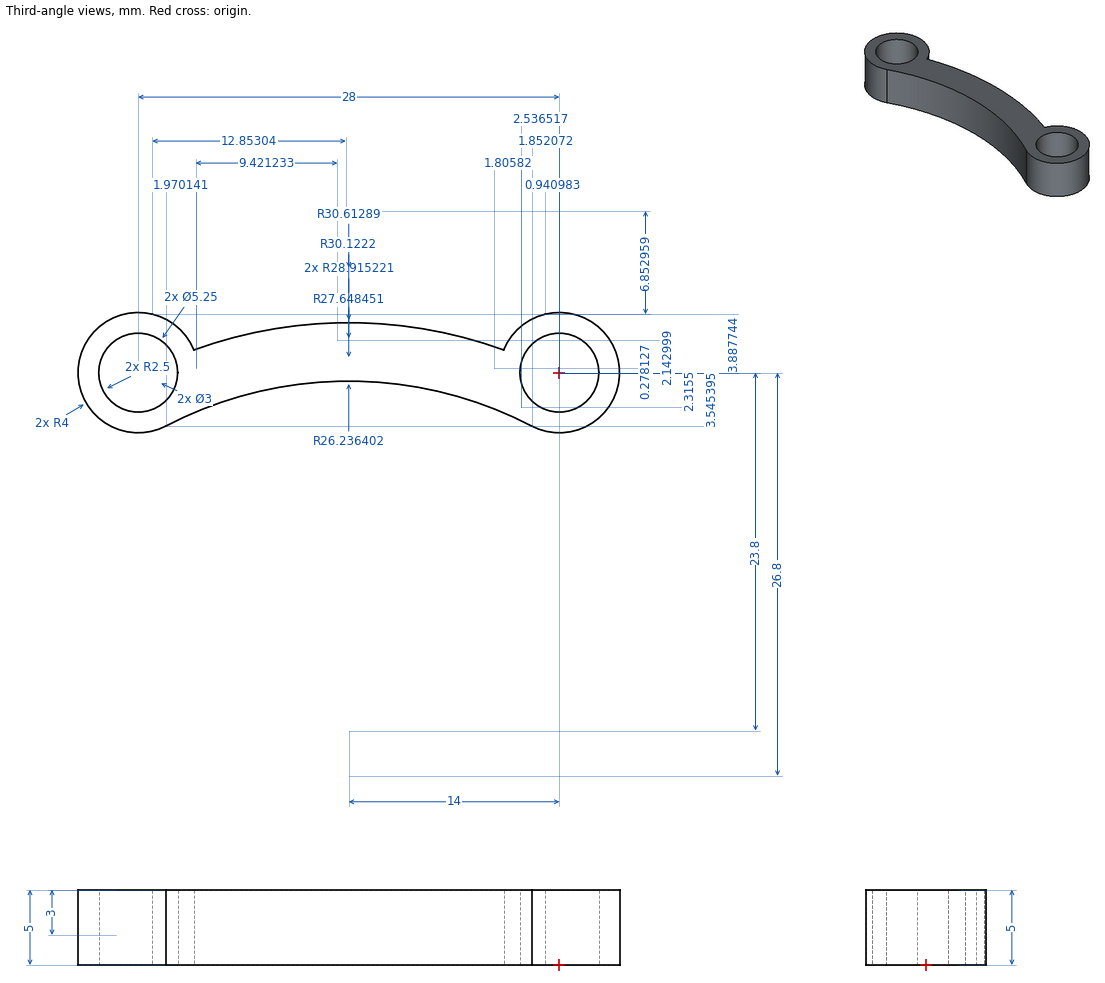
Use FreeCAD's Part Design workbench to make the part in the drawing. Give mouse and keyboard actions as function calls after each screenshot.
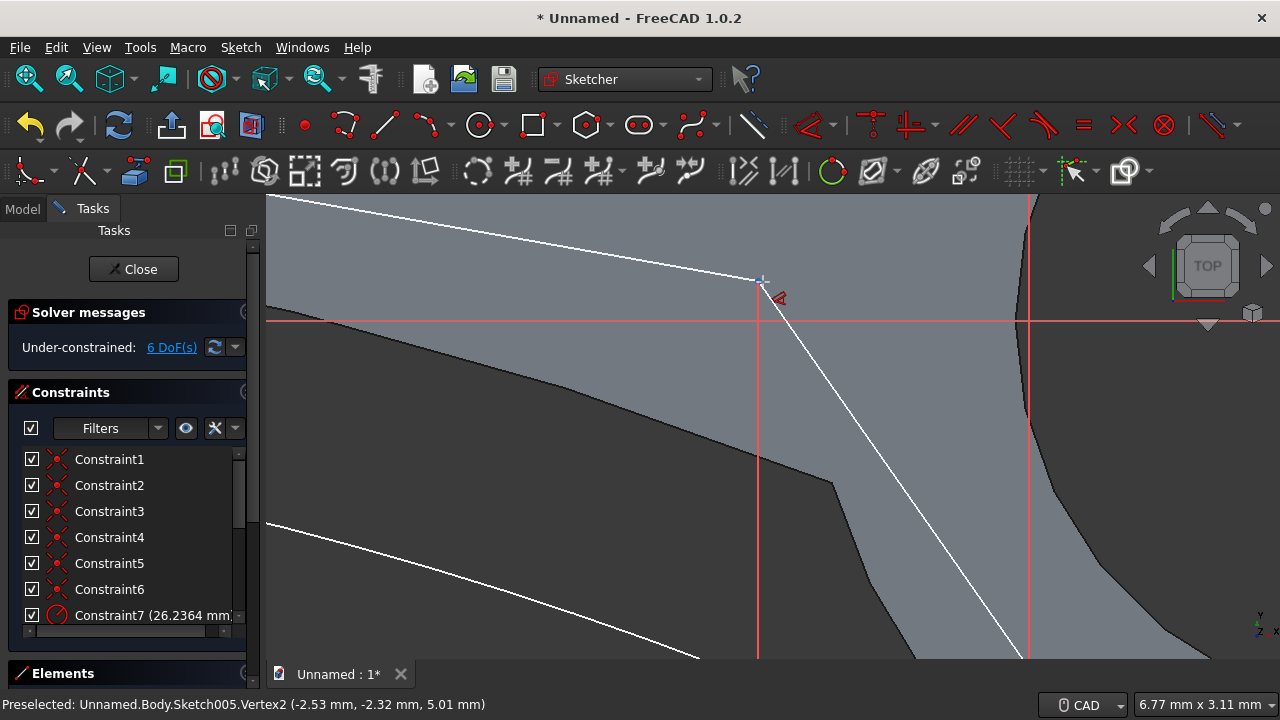
click(758, 281)
click(724, 301)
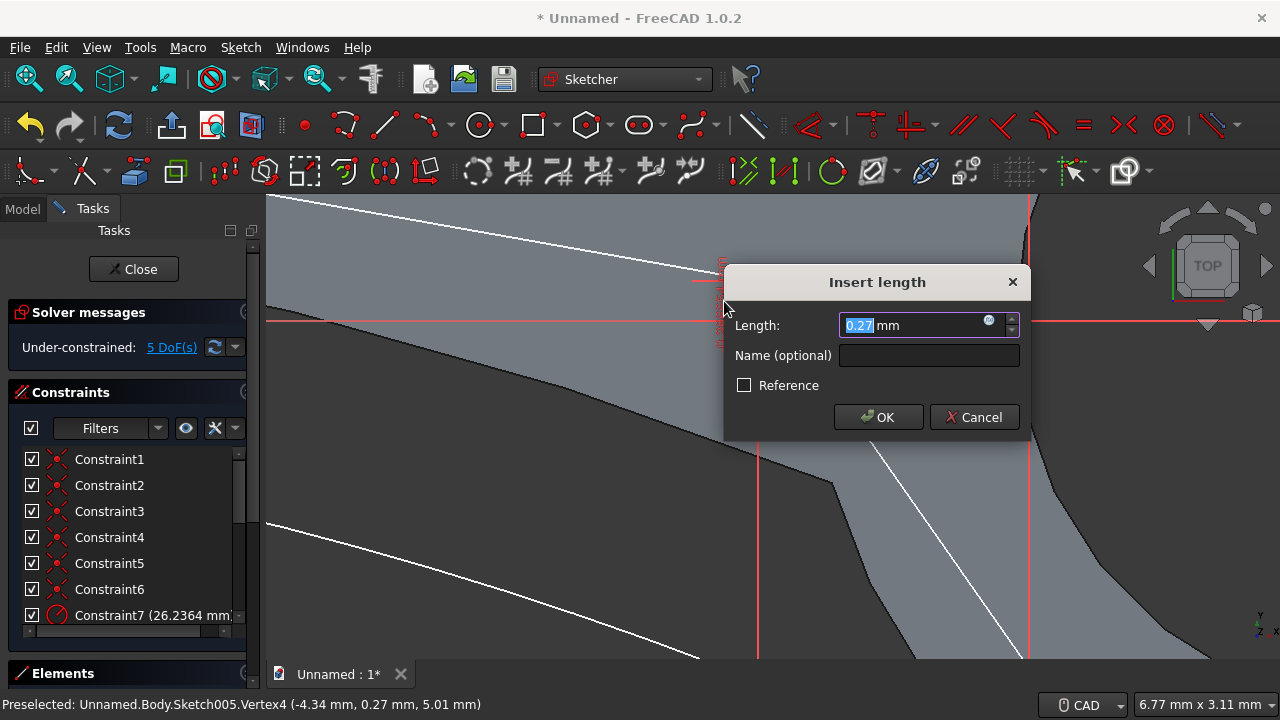
text(0.278127)
key(Return)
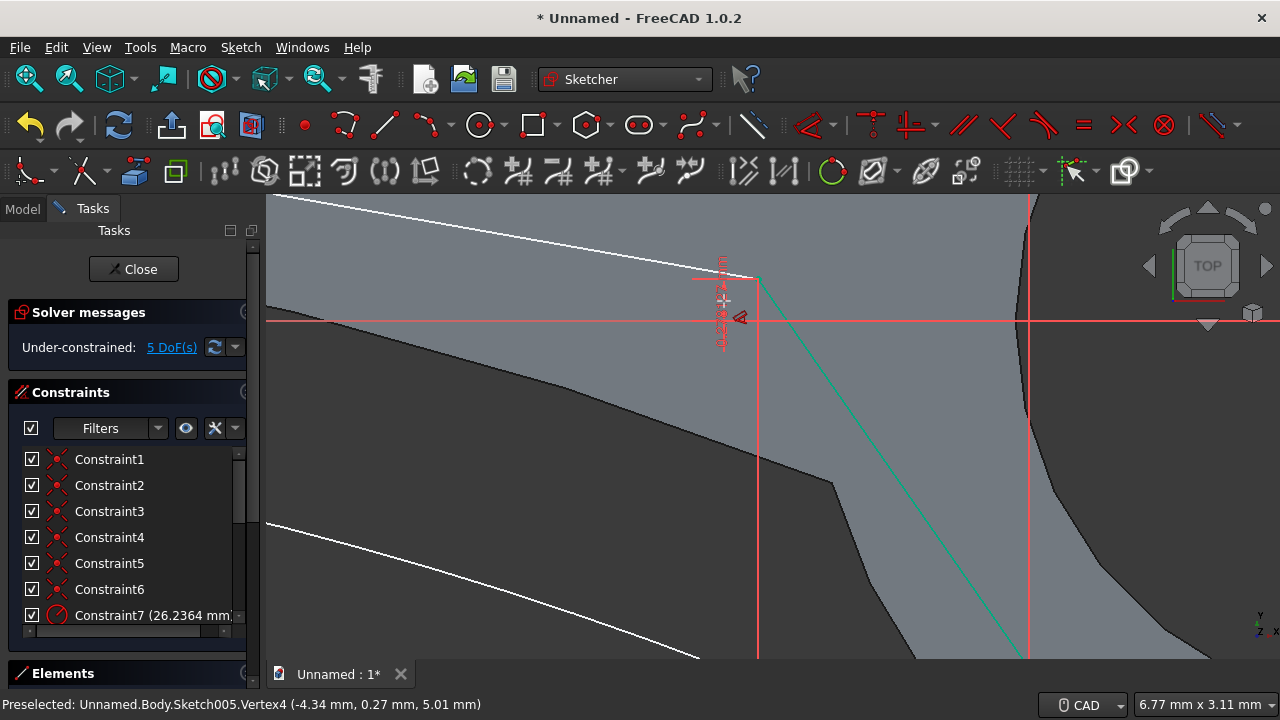
scroll(901, 427, down, 10)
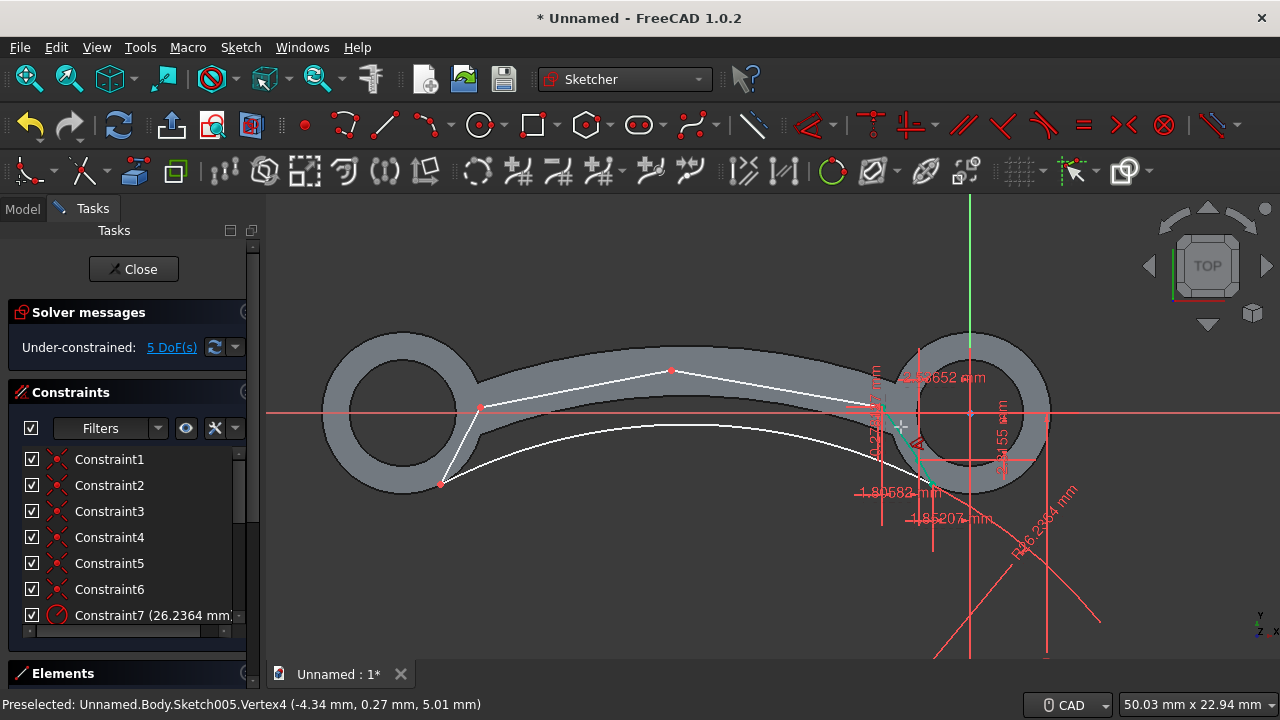
click(671, 370)
click(637, 392)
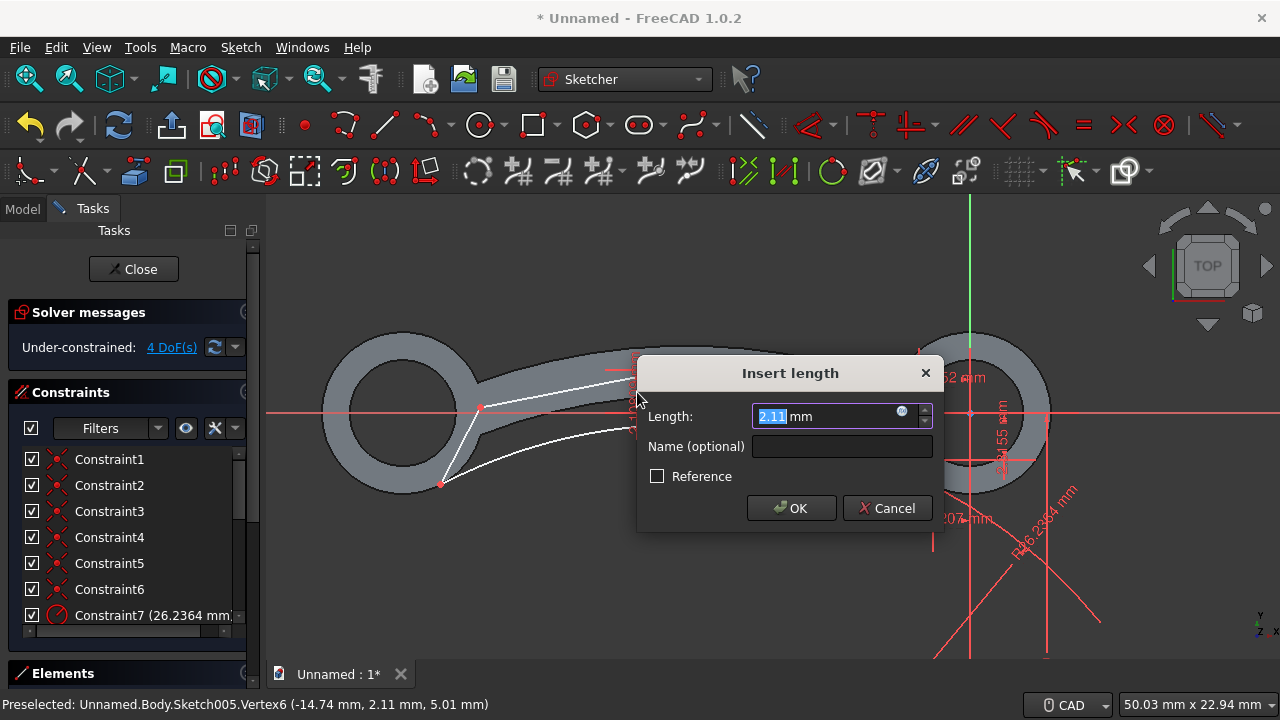
text(2.142999)
key(Return)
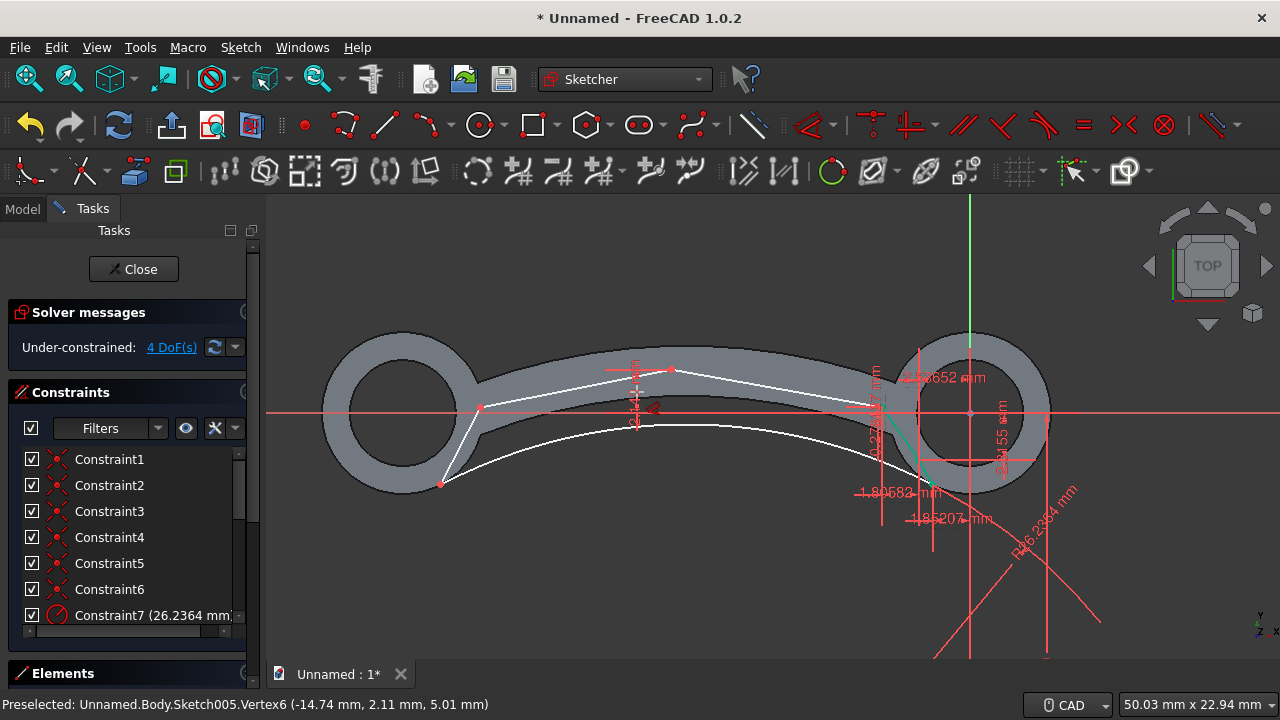
scroll(480, 408, up, 10)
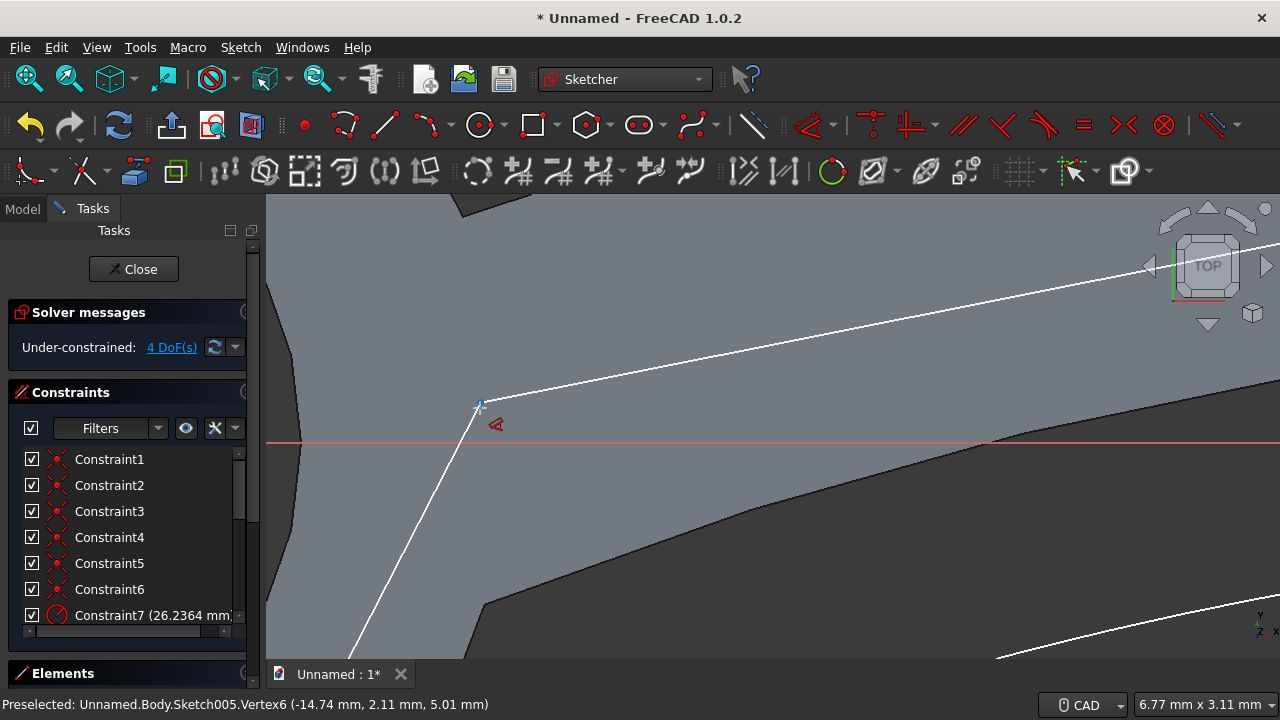
click(481, 403)
click(447, 423)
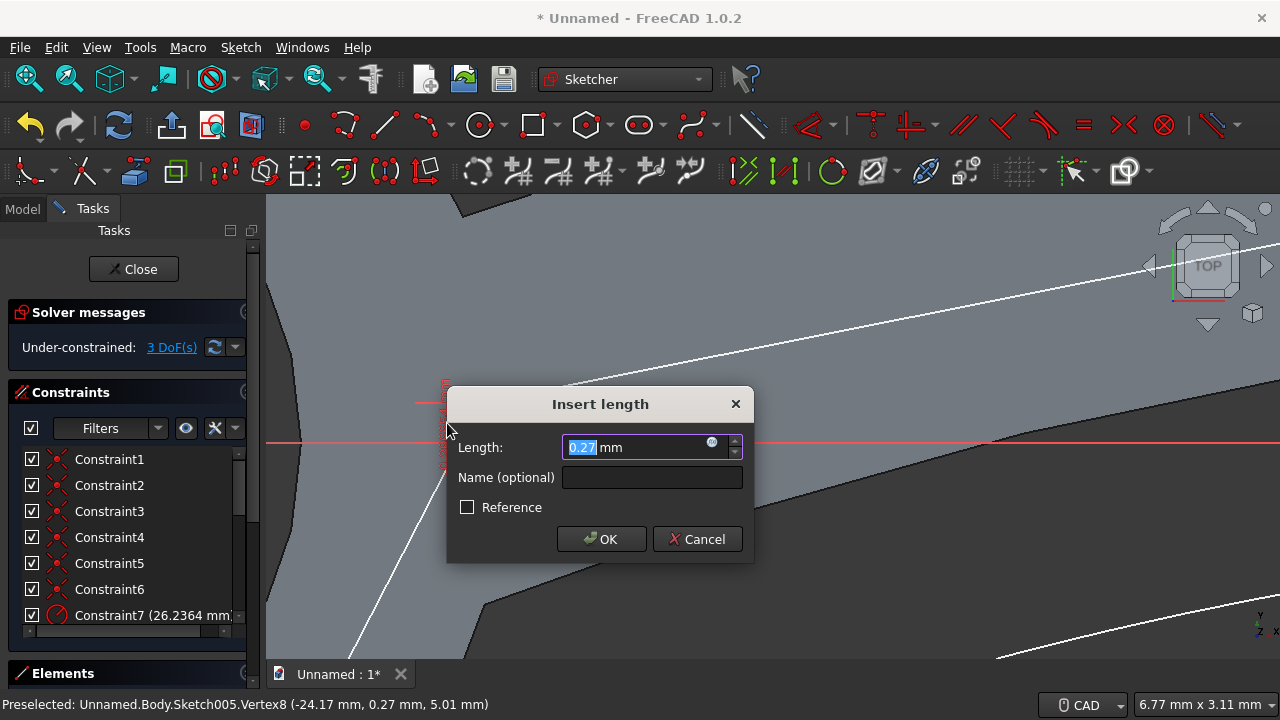
text(0.278127)
key(Return)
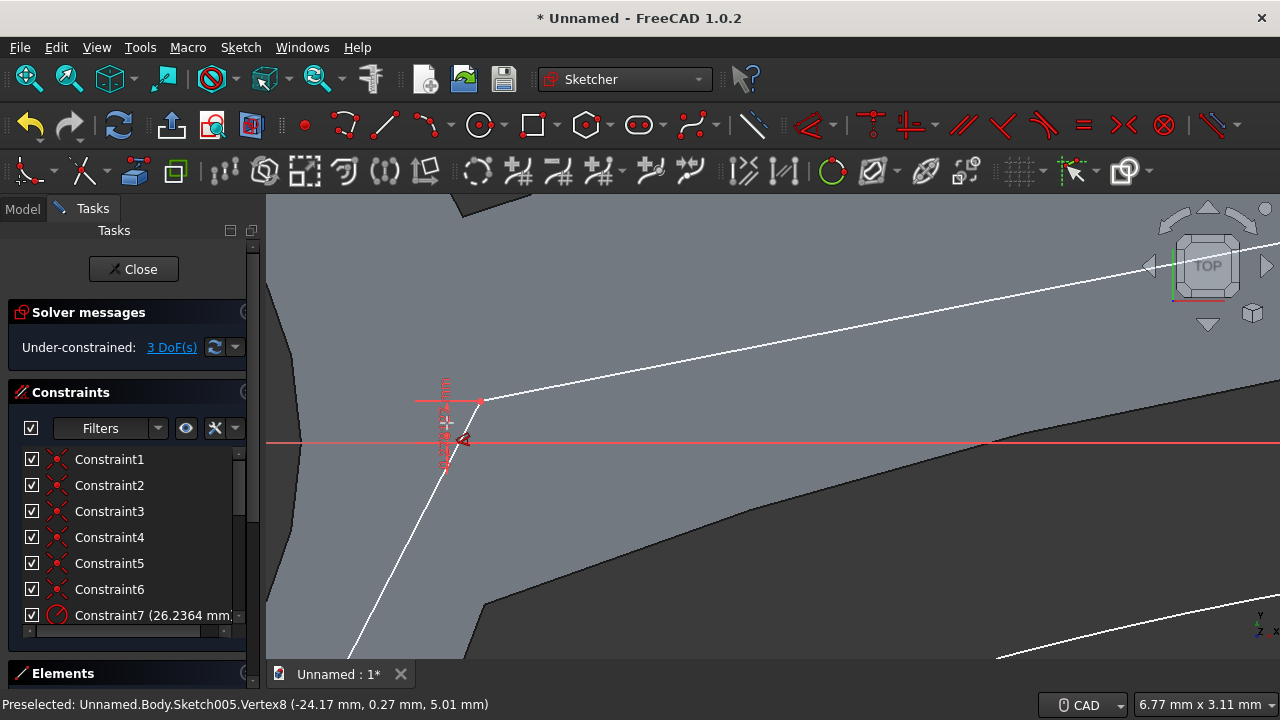
scroll(479, 408, down, 10)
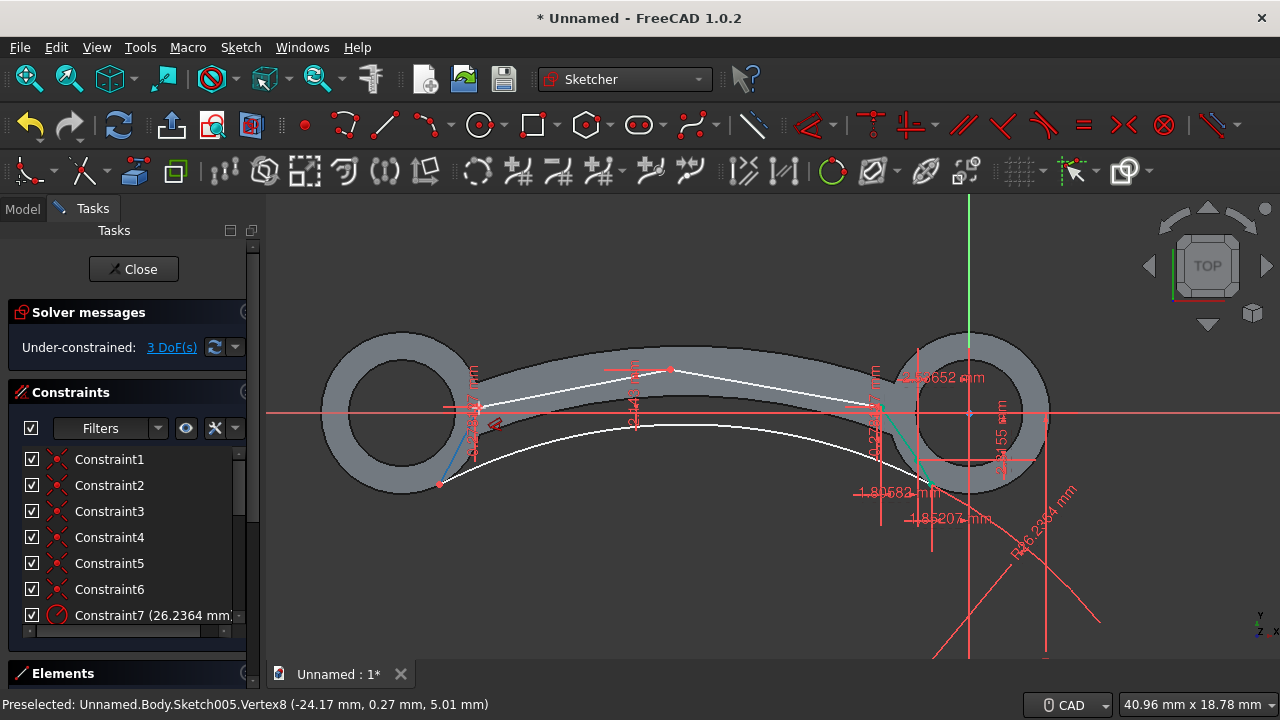
click(440, 485)
click(1003, 465)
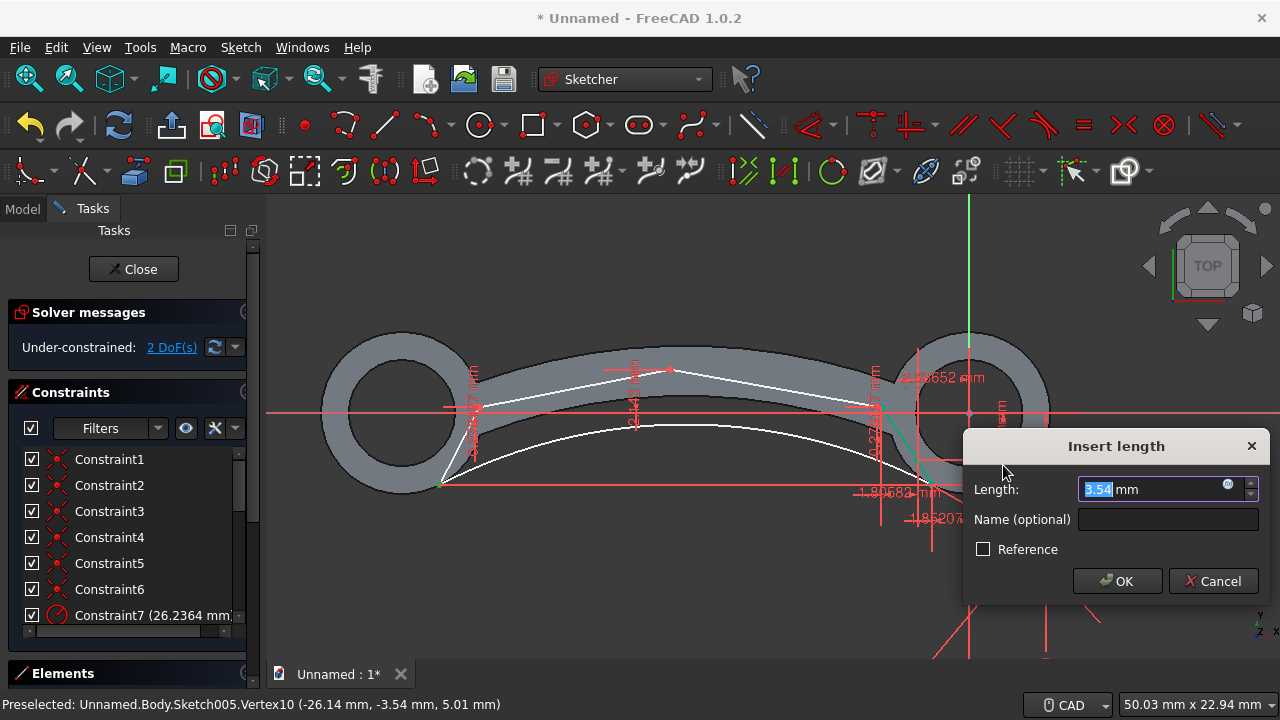
text(3.545395)
key(Return)